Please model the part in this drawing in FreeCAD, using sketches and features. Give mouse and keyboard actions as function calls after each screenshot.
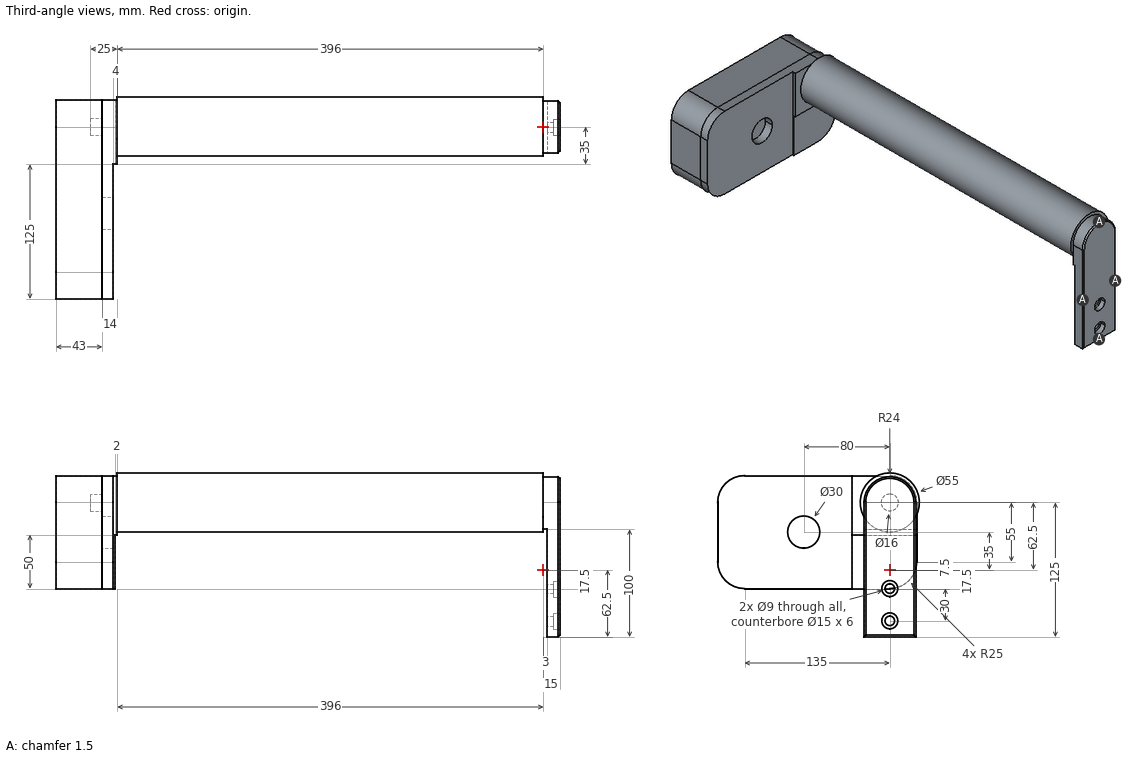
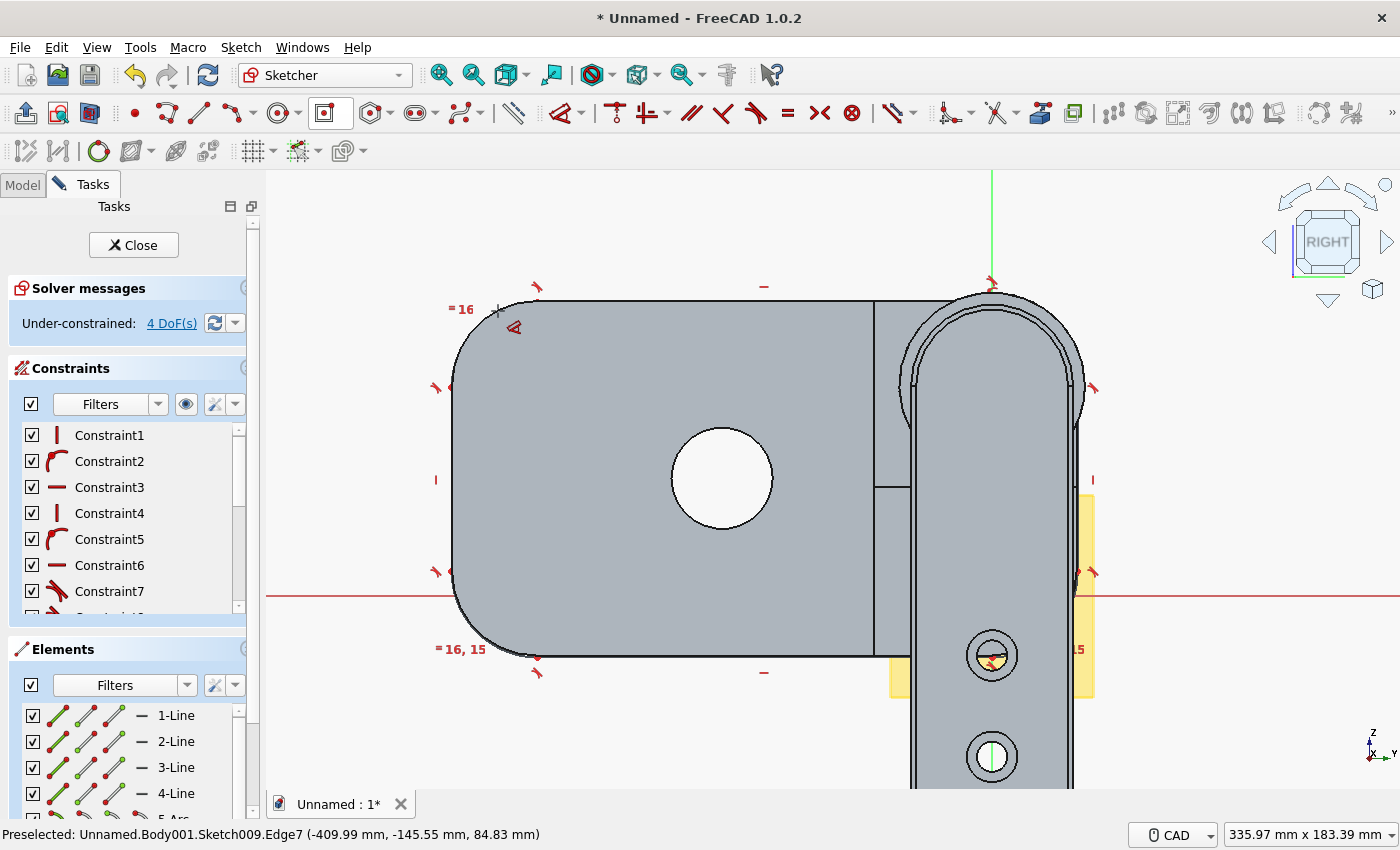
click(1031, 648)
click(1046, 676)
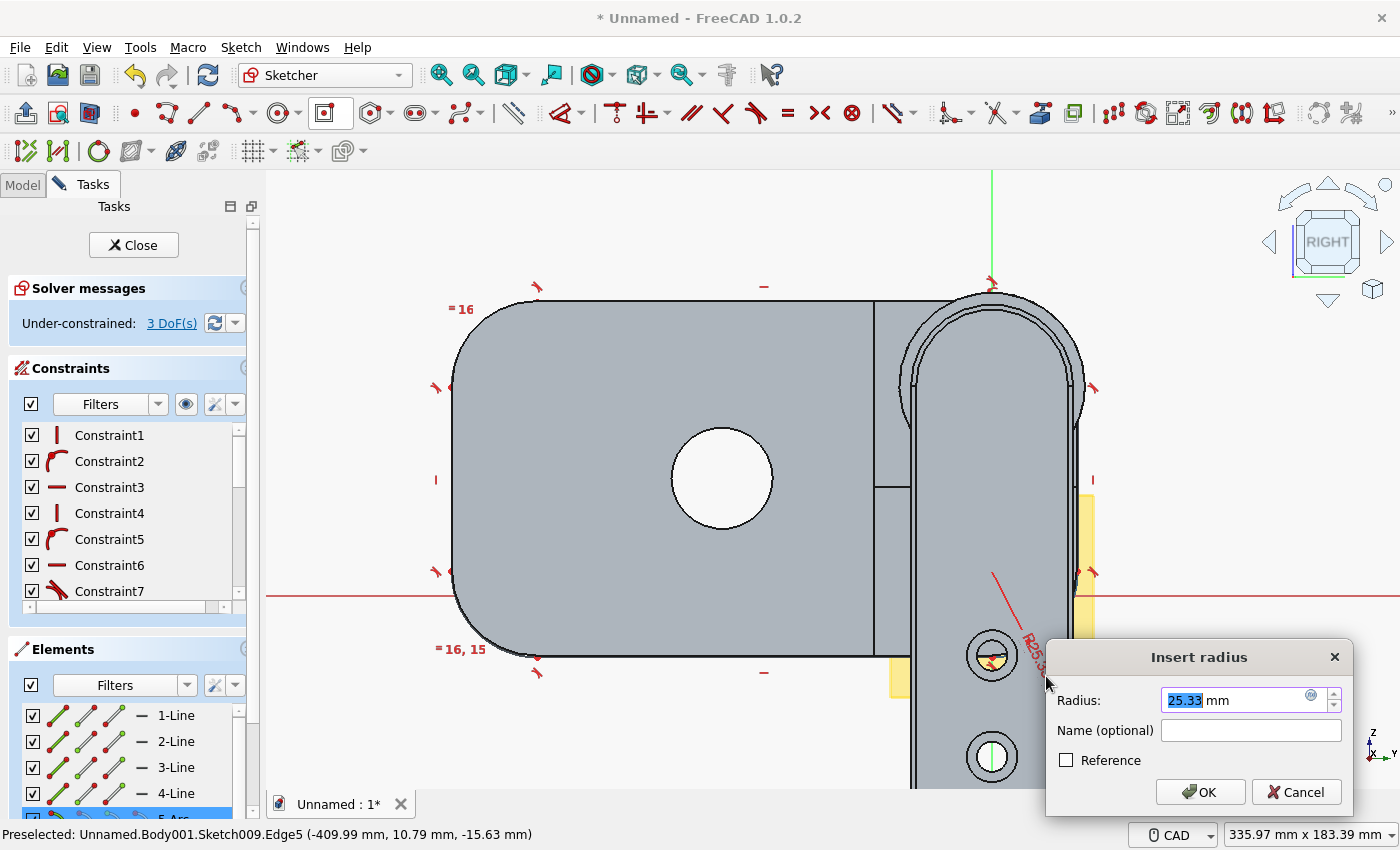
text(25)
key(Return)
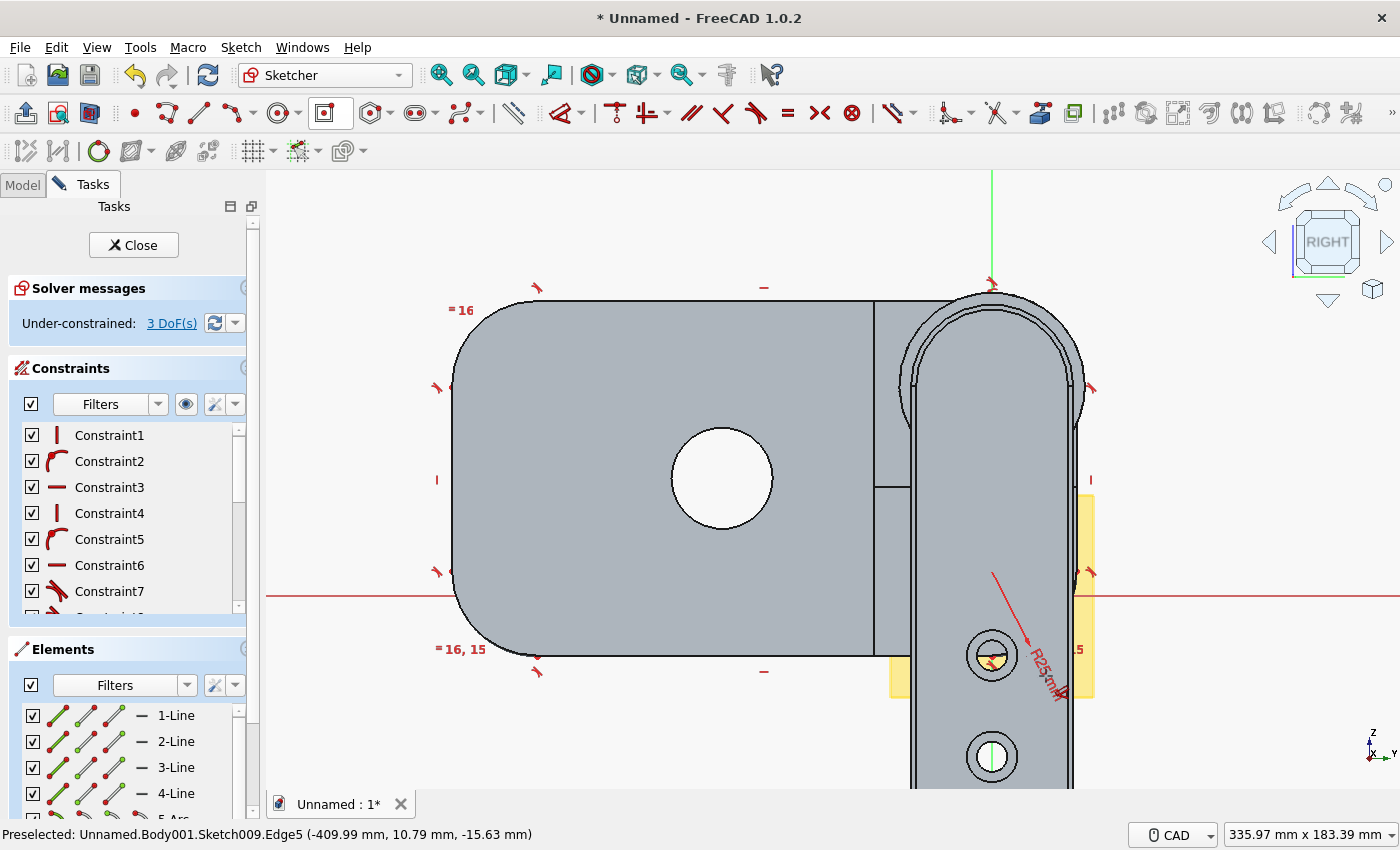
click(1077, 443)
click(1111, 480)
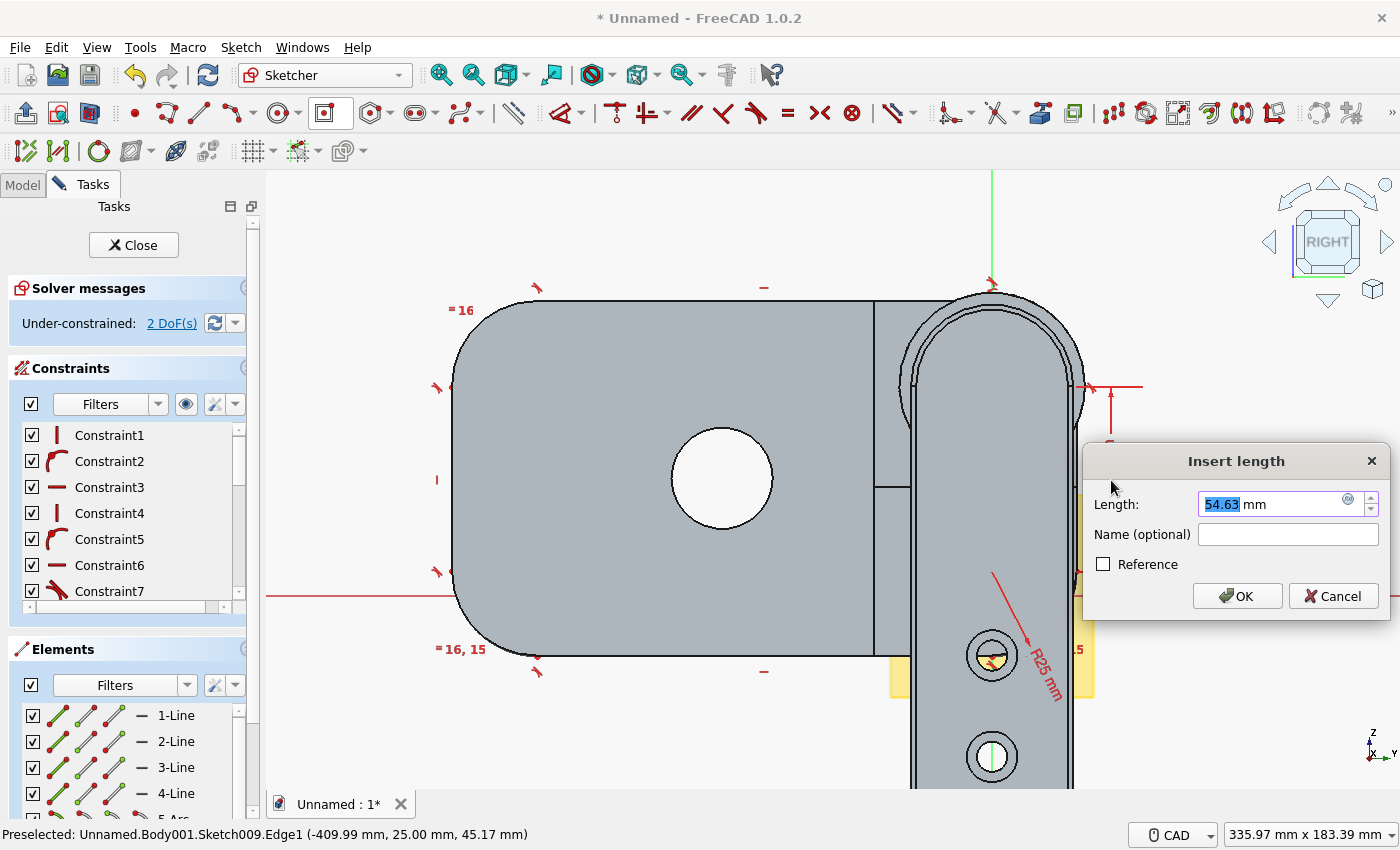
text(55)
key(Return)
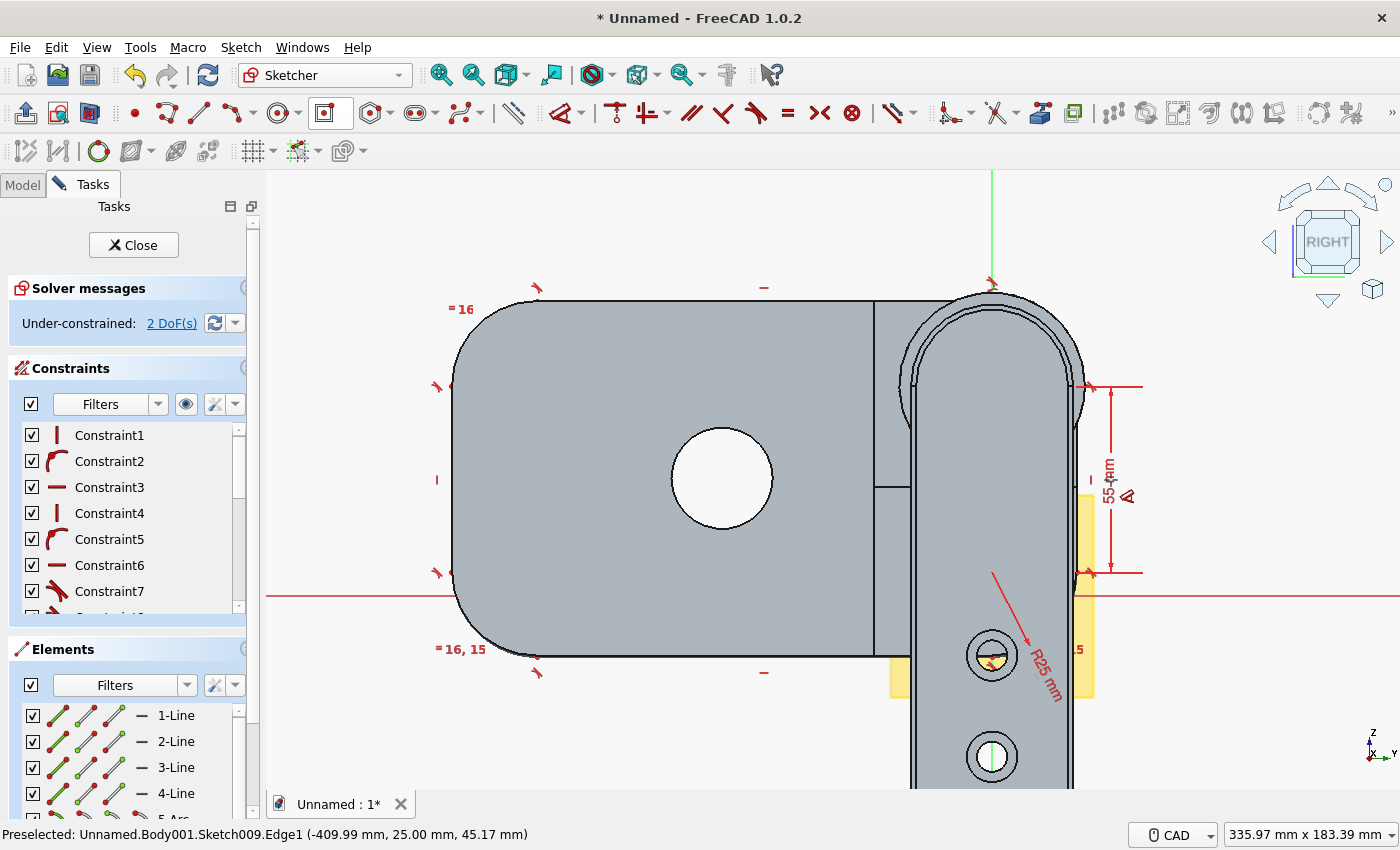
click(856, 657)
click(765, 691)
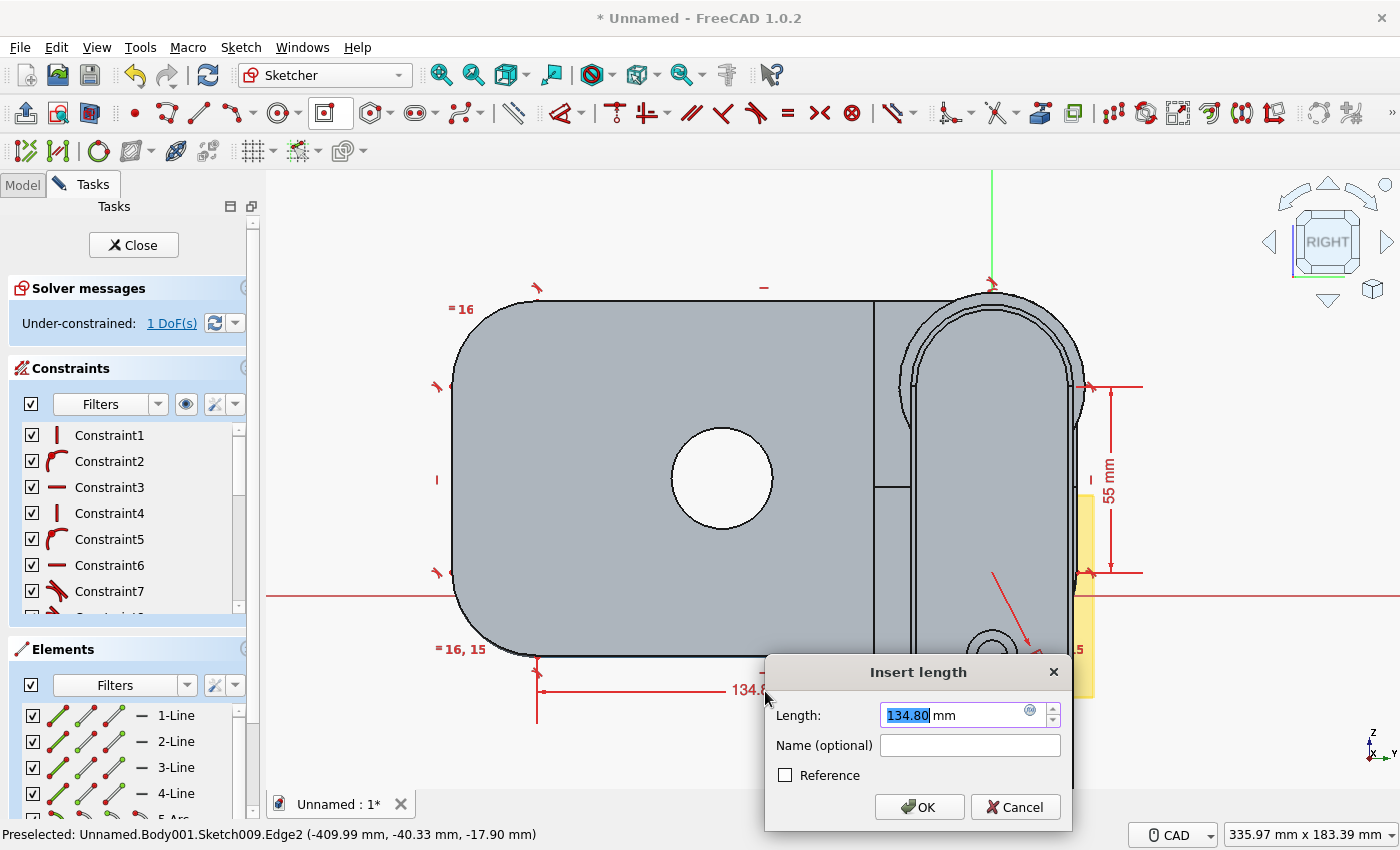
text(135)
key(Return)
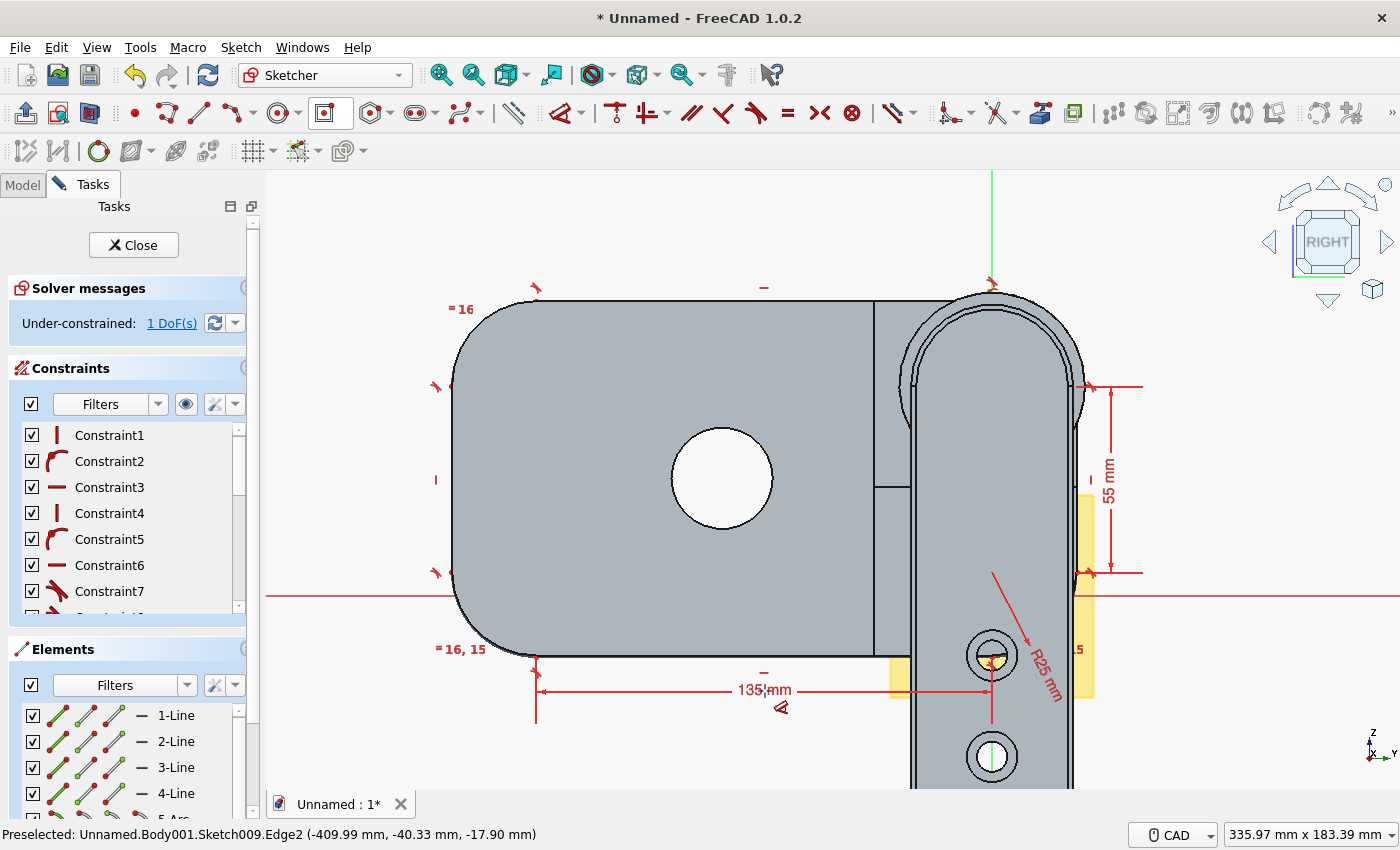
scroll(1077, 573, up, 3)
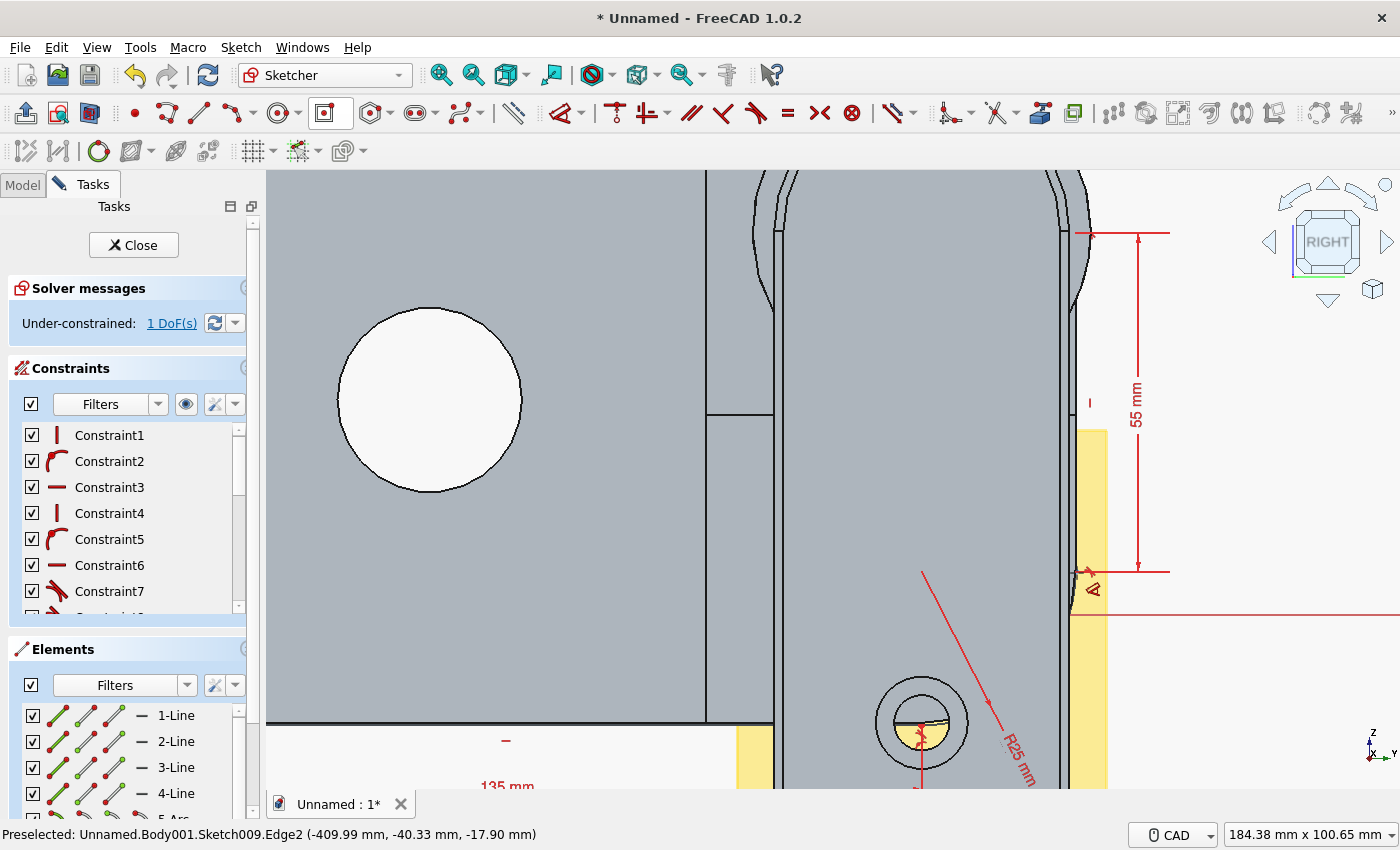
click(1076, 572)
click(1110, 593)